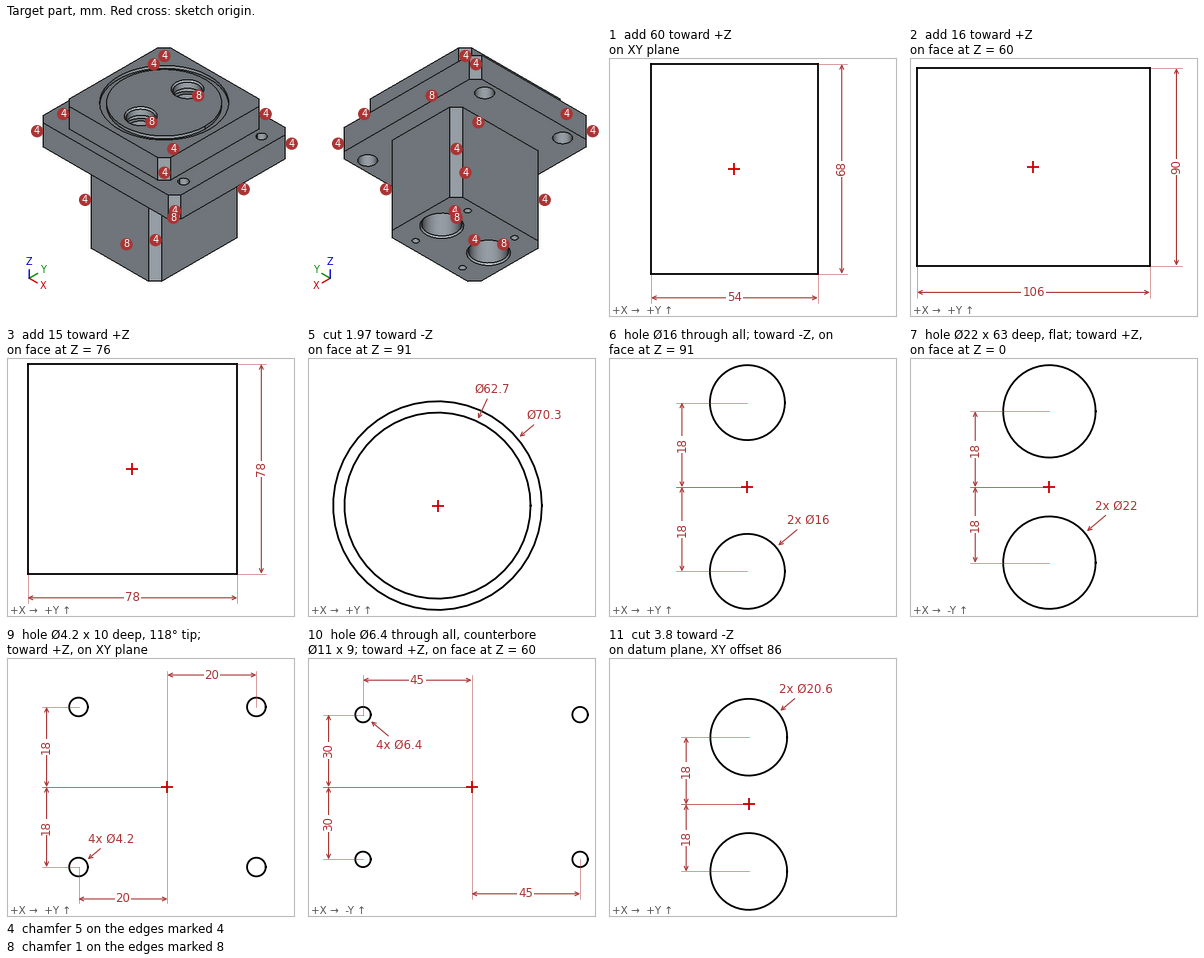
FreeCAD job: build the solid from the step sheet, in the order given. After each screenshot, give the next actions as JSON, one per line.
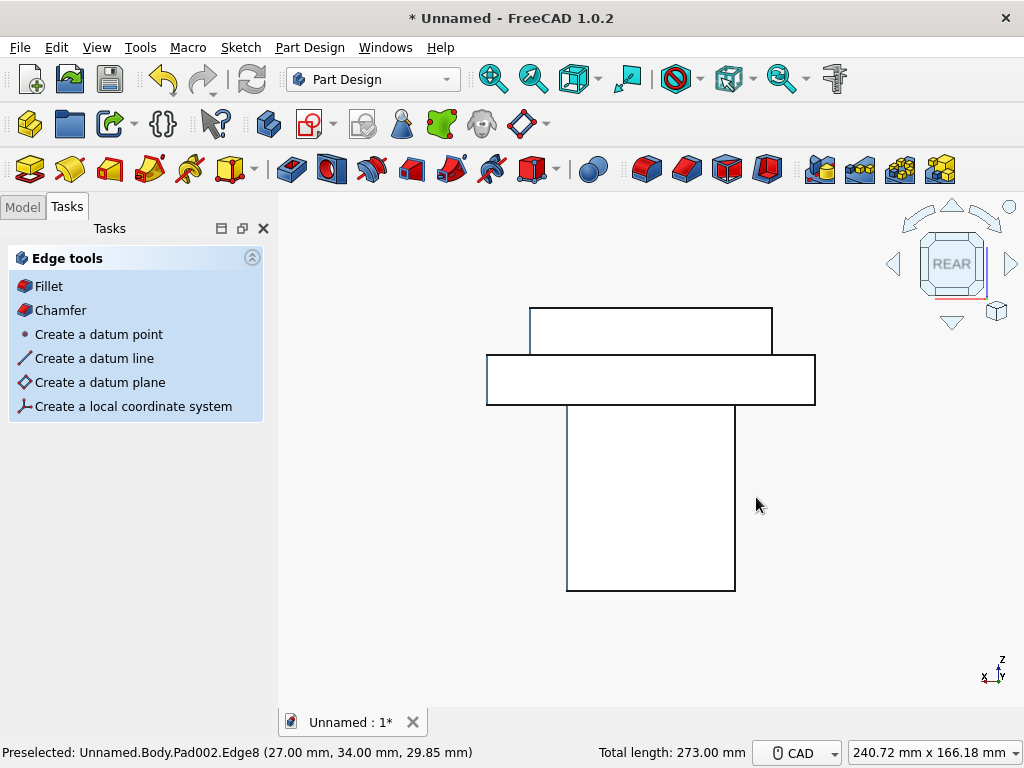
{"action": "left_click", "coordinate": [815, 379], "text": "ctrl"}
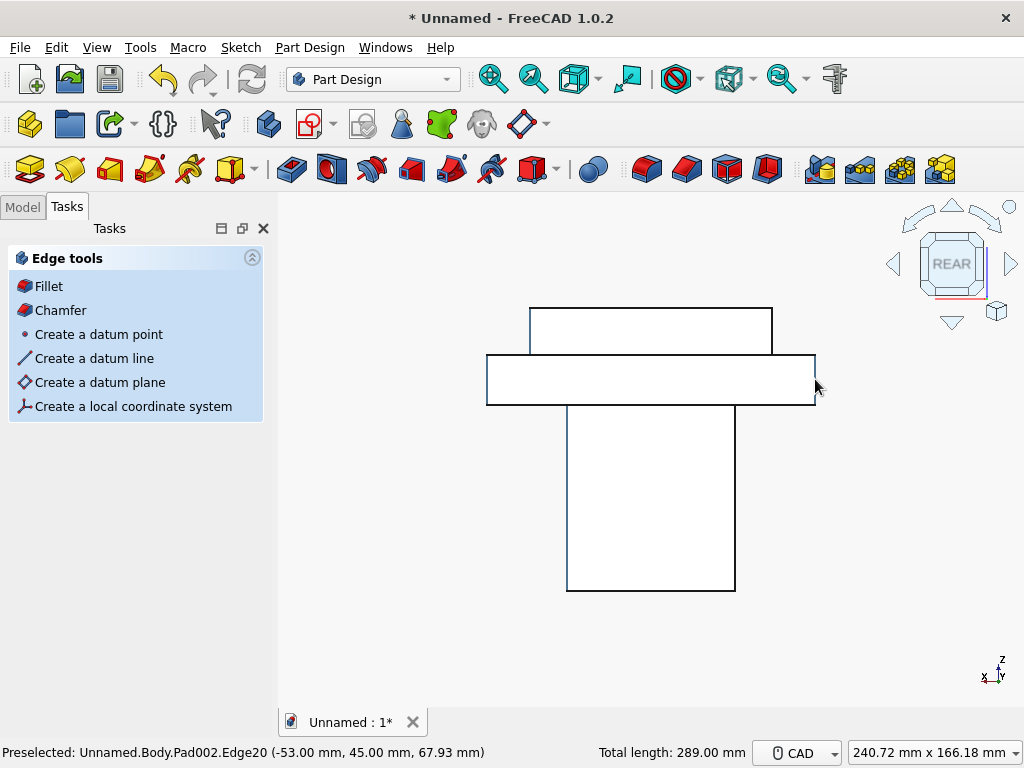
{"action": "left_click", "coordinate": [772, 331], "text": "ctrl"}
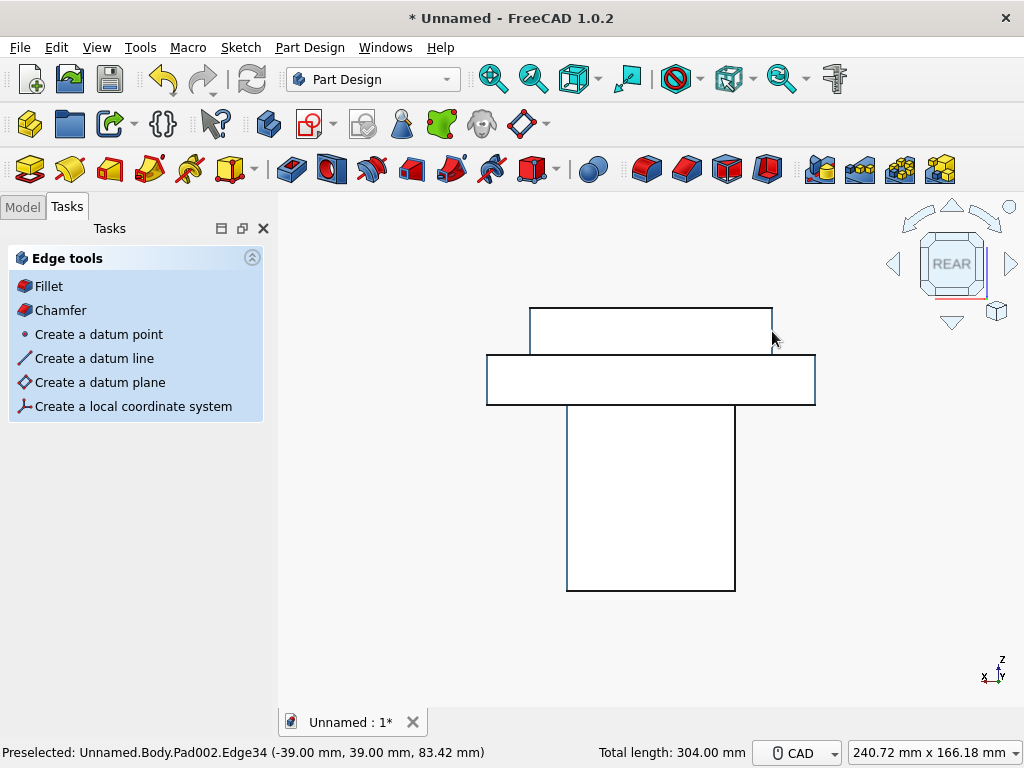
{"action": "left_click", "coordinate": [735, 497], "text": "ctrl"}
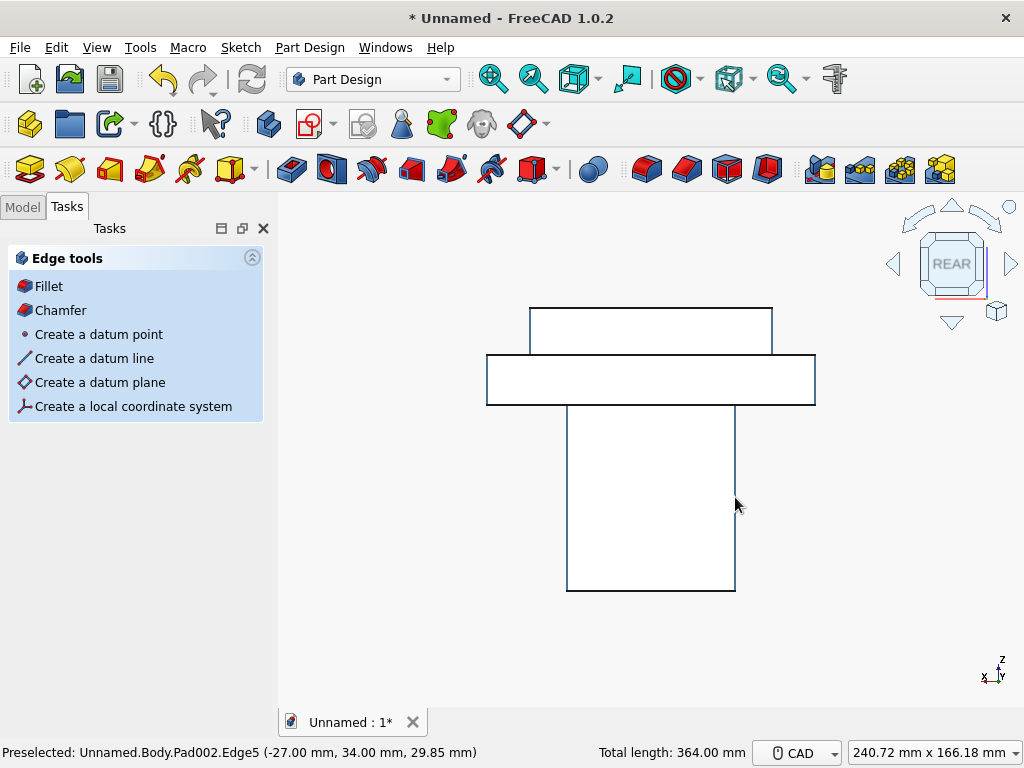
{"action": "left_click", "coordinate": [688, 170]}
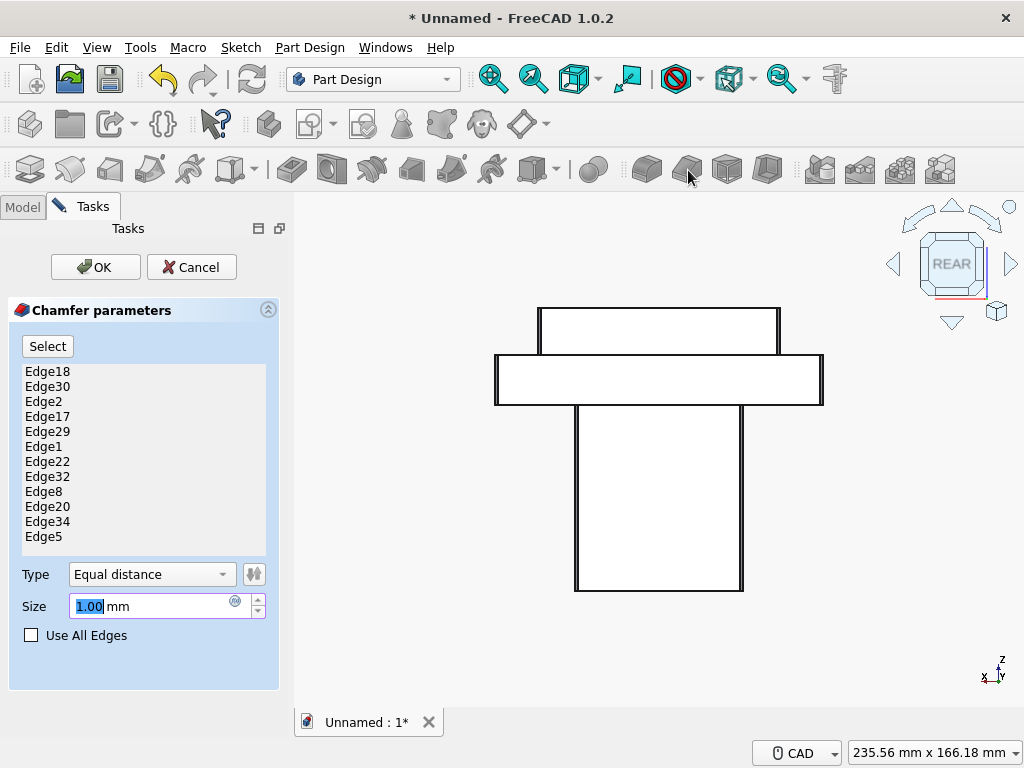
{"action": "type", "text": "5"}
{"action": "key", "text": "Tab"}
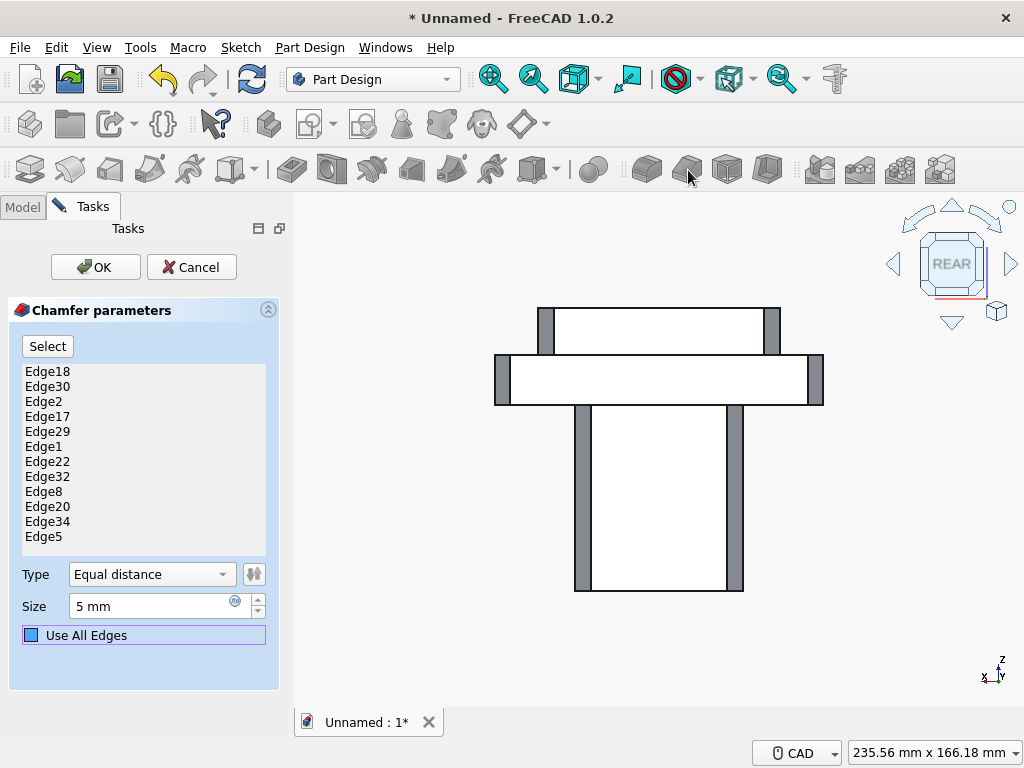
{"action": "left_click", "coordinate": [96, 267]}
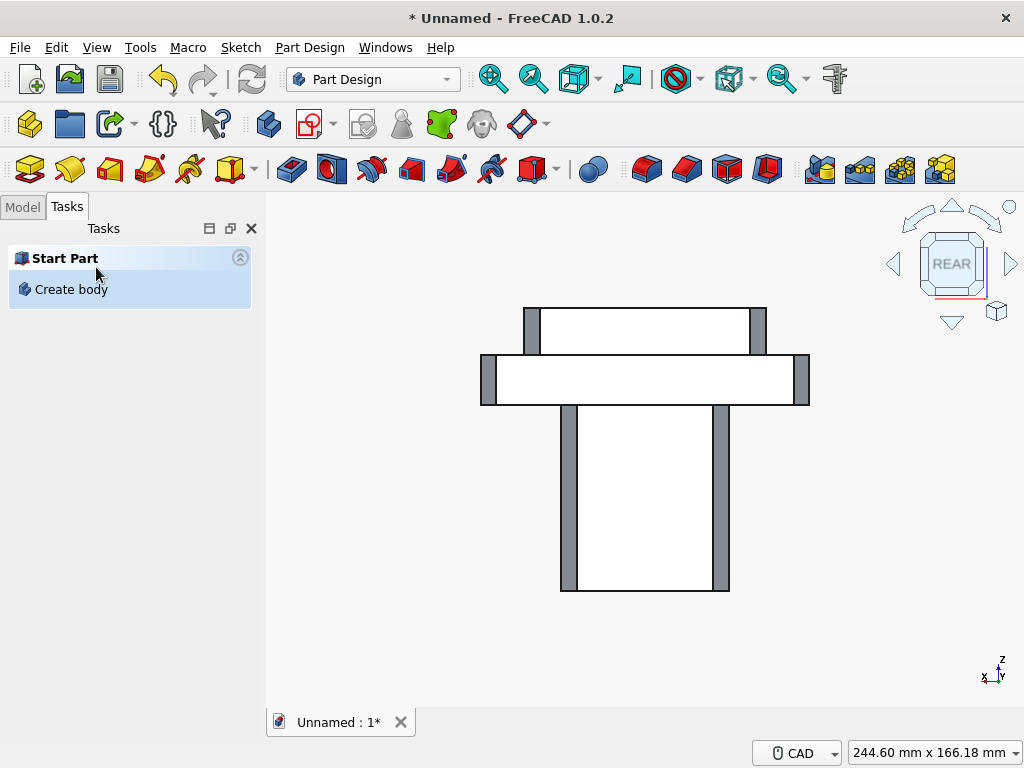
{"action": "key", "text": "0"}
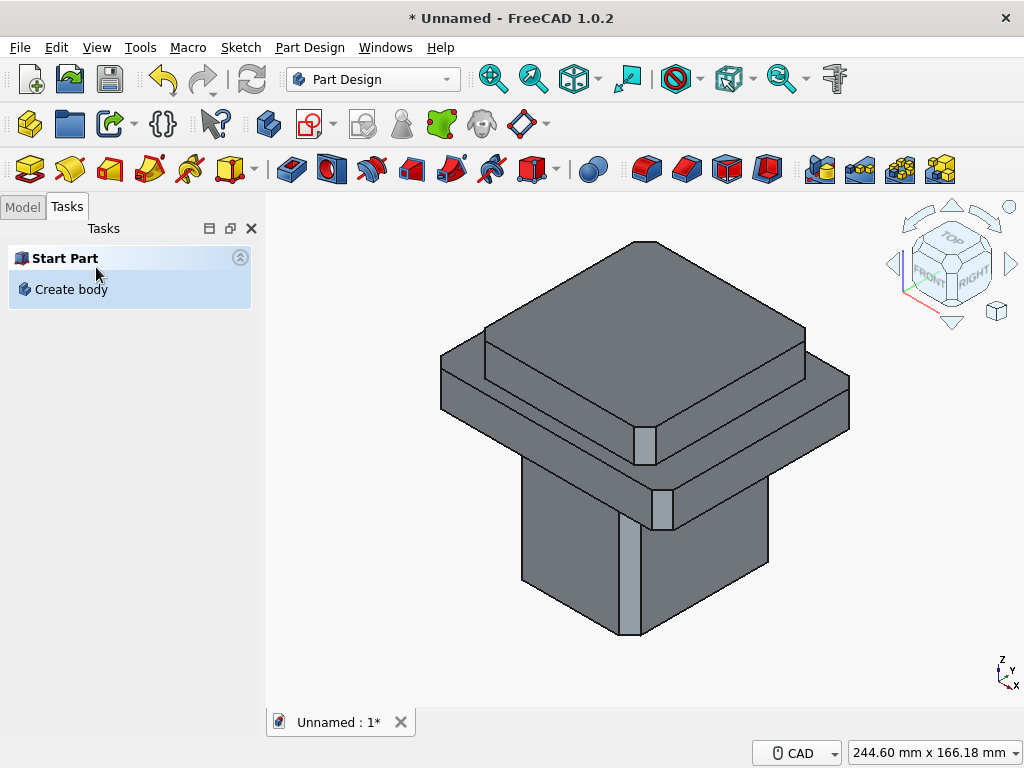
{"action": "left_click", "coordinate": [645, 333]}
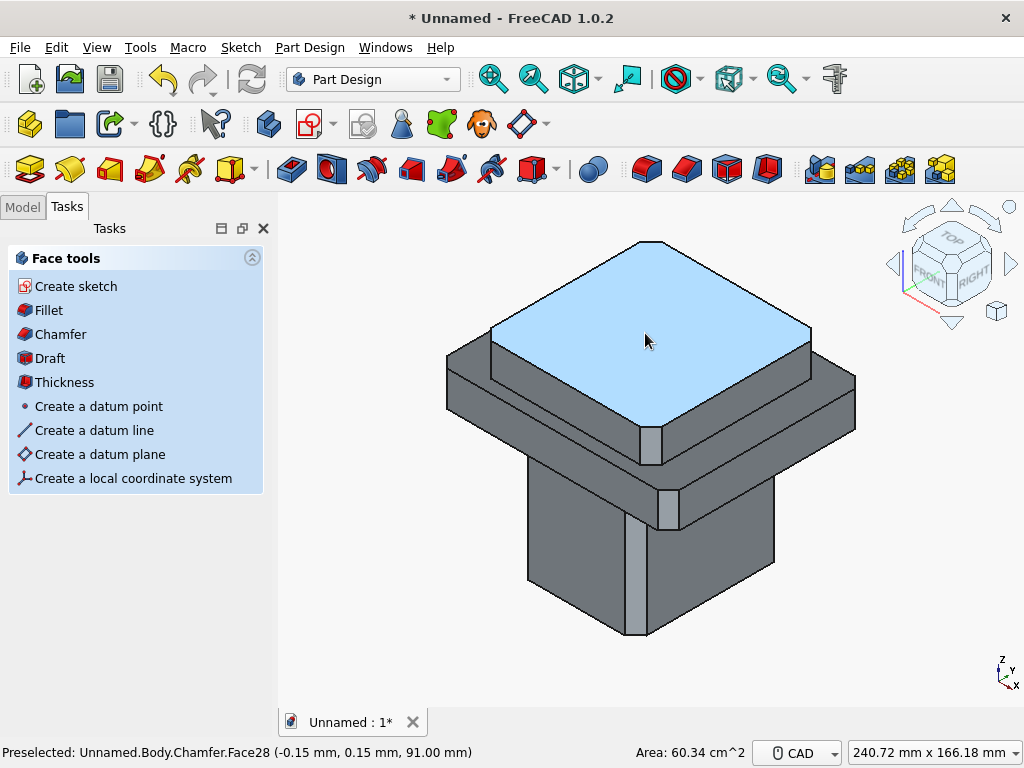
{"action": "left_click", "coordinate": [310, 124]}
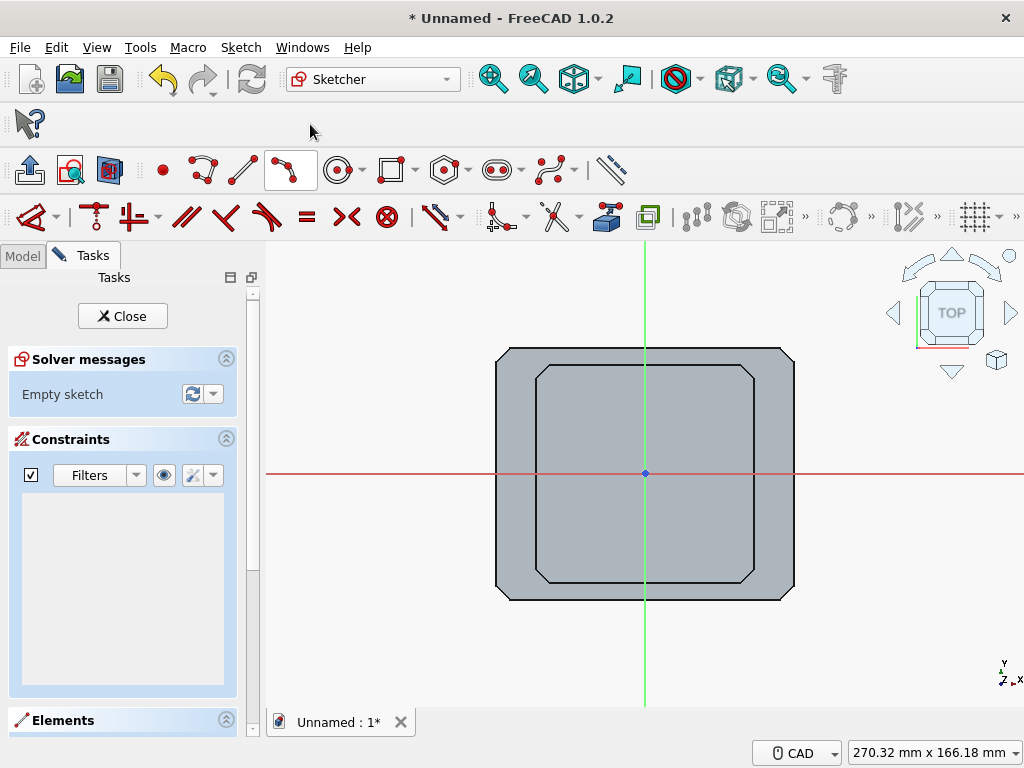
{"action": "scroll", "coordinate": [784, 474], "scroll_direction": "up", "scroll_amount": 2}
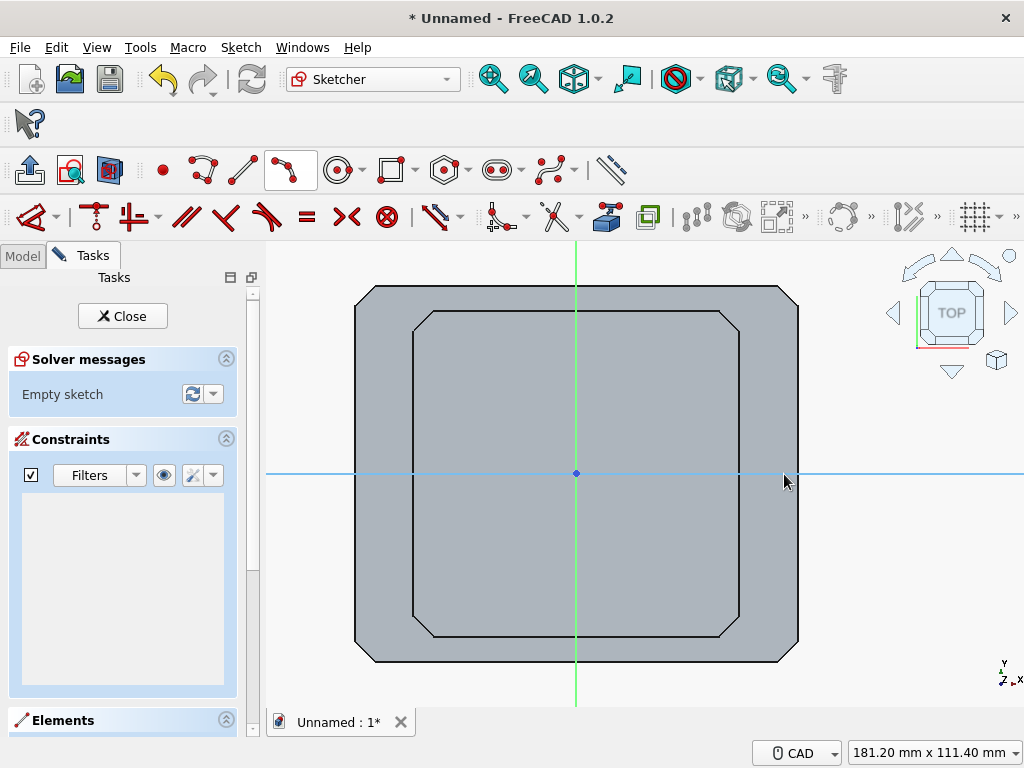
{"action": "key", "text": "g c"}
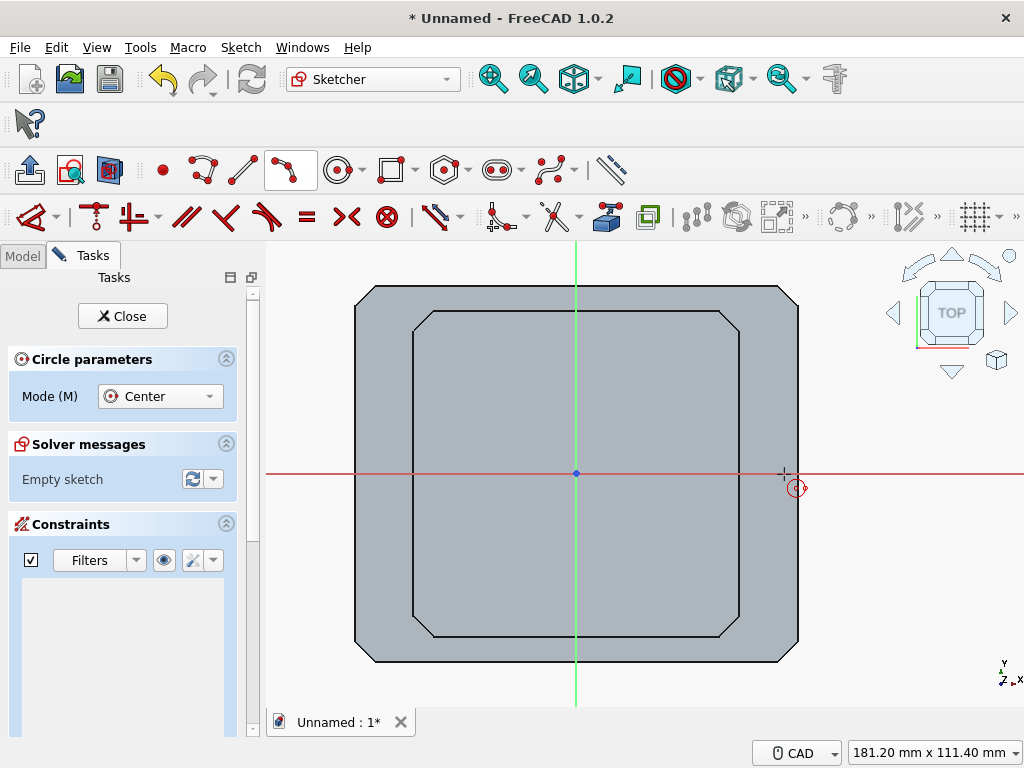
{"action": "left_click", "coordinate": [576, 474]}
{"action": "mouse_move", "coordinate": [680, 370]}